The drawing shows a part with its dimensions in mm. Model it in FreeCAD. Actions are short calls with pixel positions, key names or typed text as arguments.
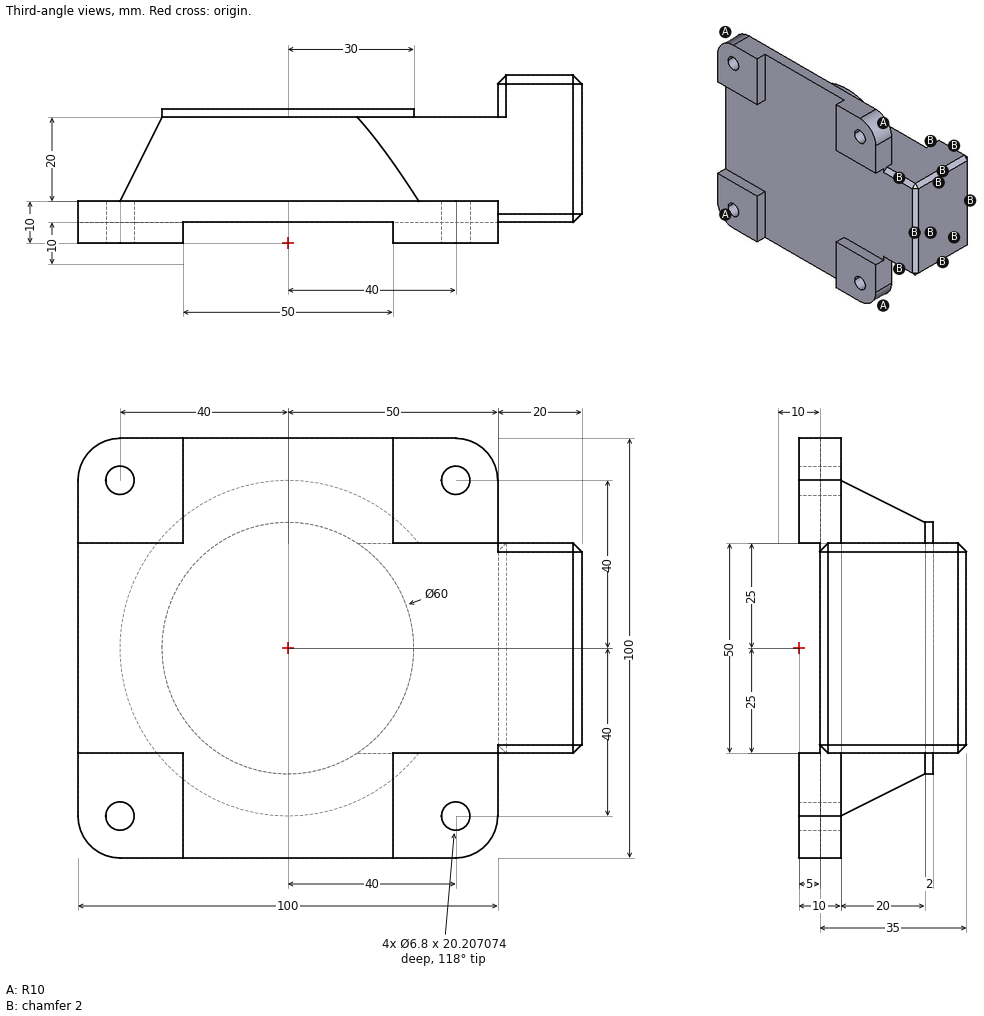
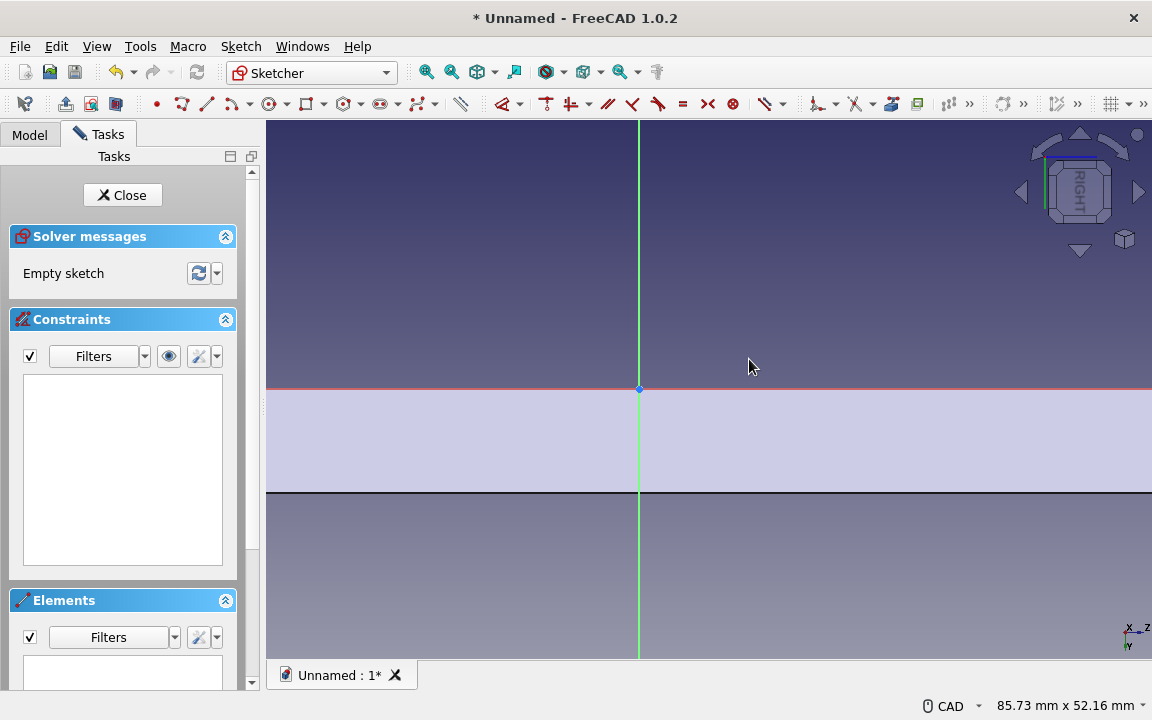
key(g)
key(v)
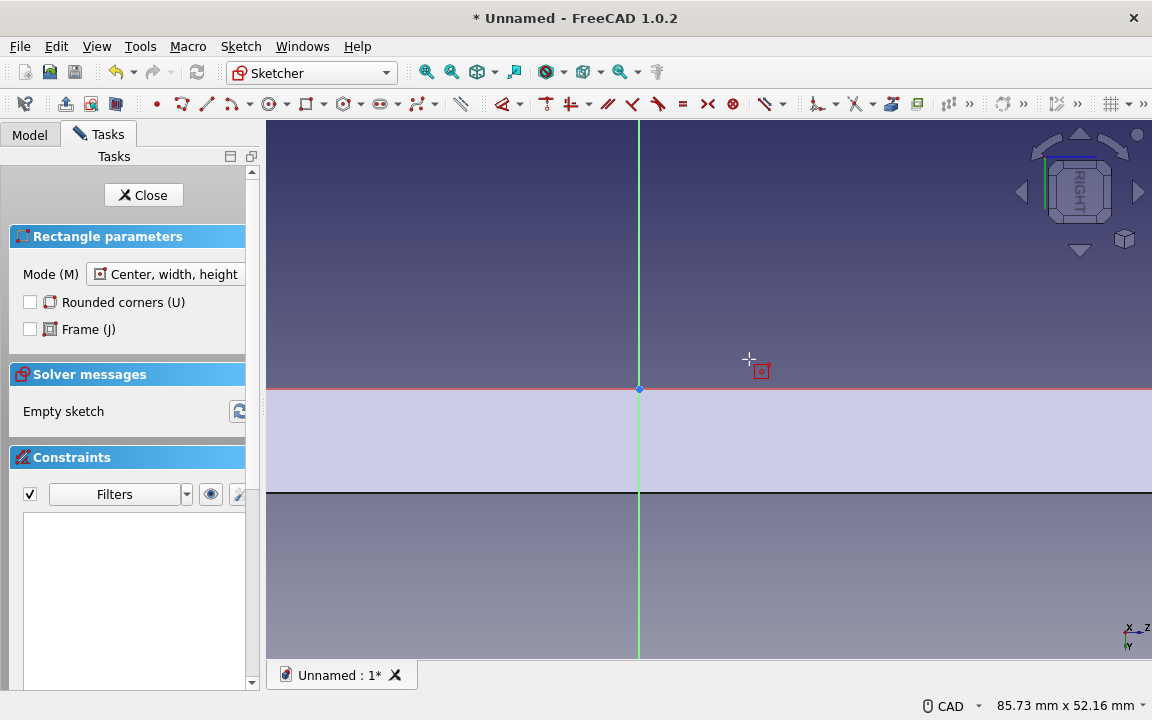
click(639, 389)
click(898, 338)
key(Escape)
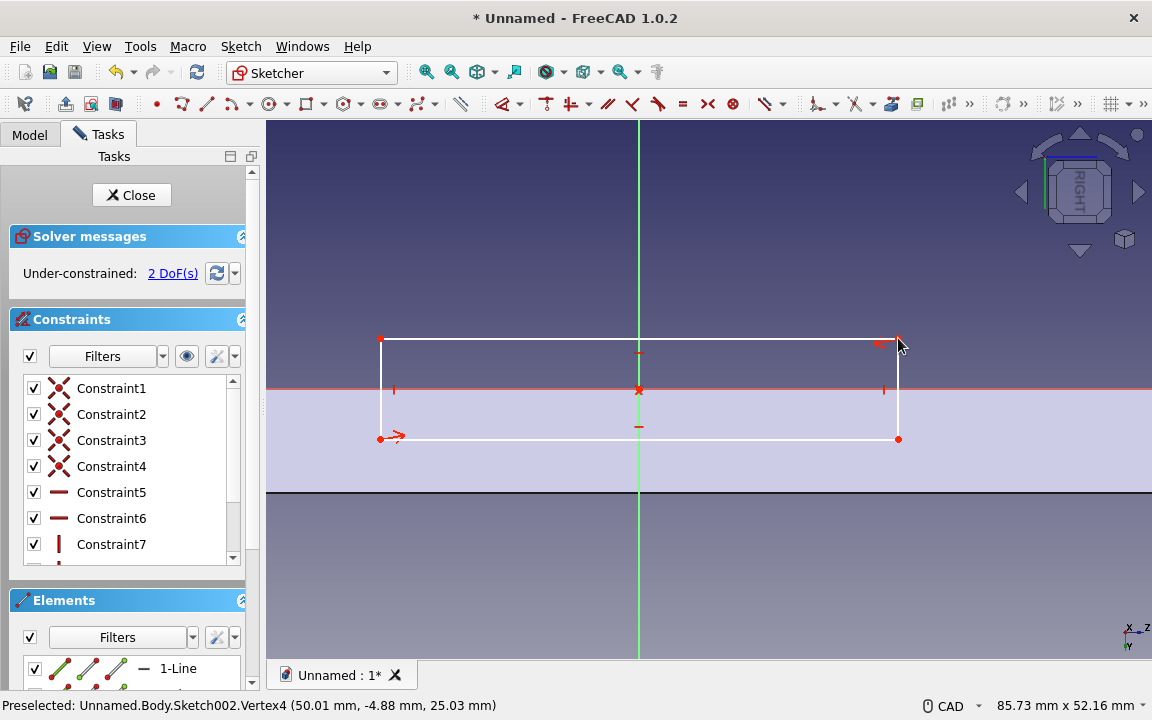
click(502, 104)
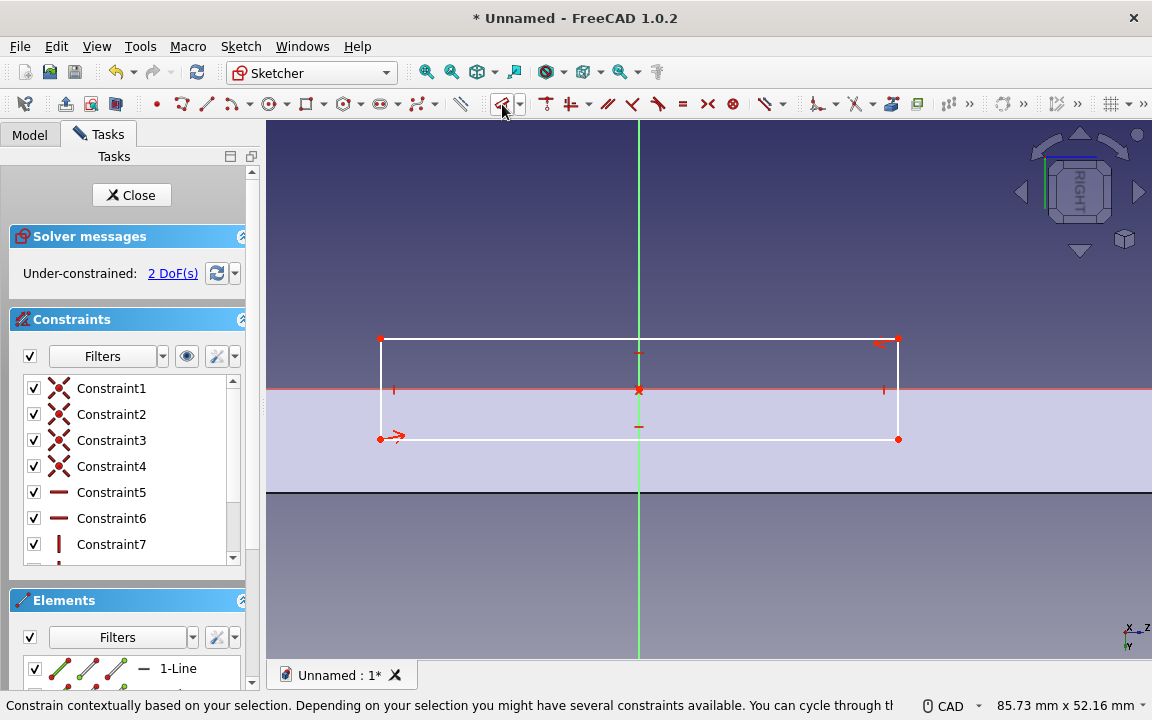
click(536, 440)
click(520, 474)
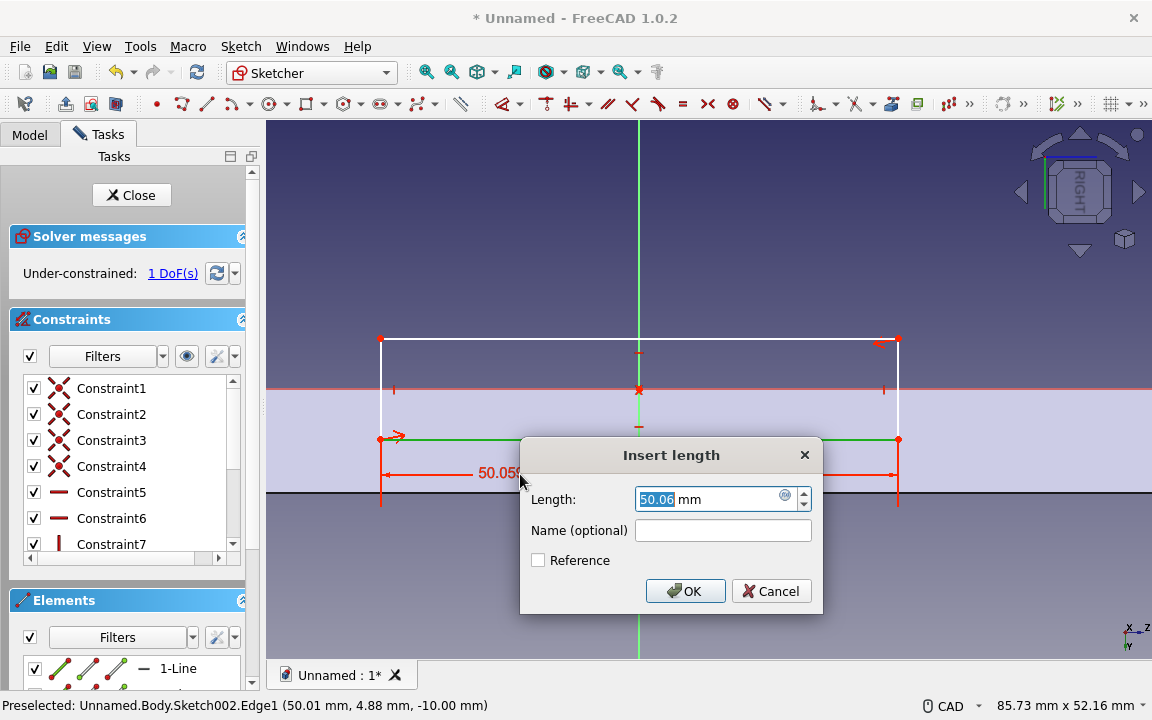
text(50)
key(Return)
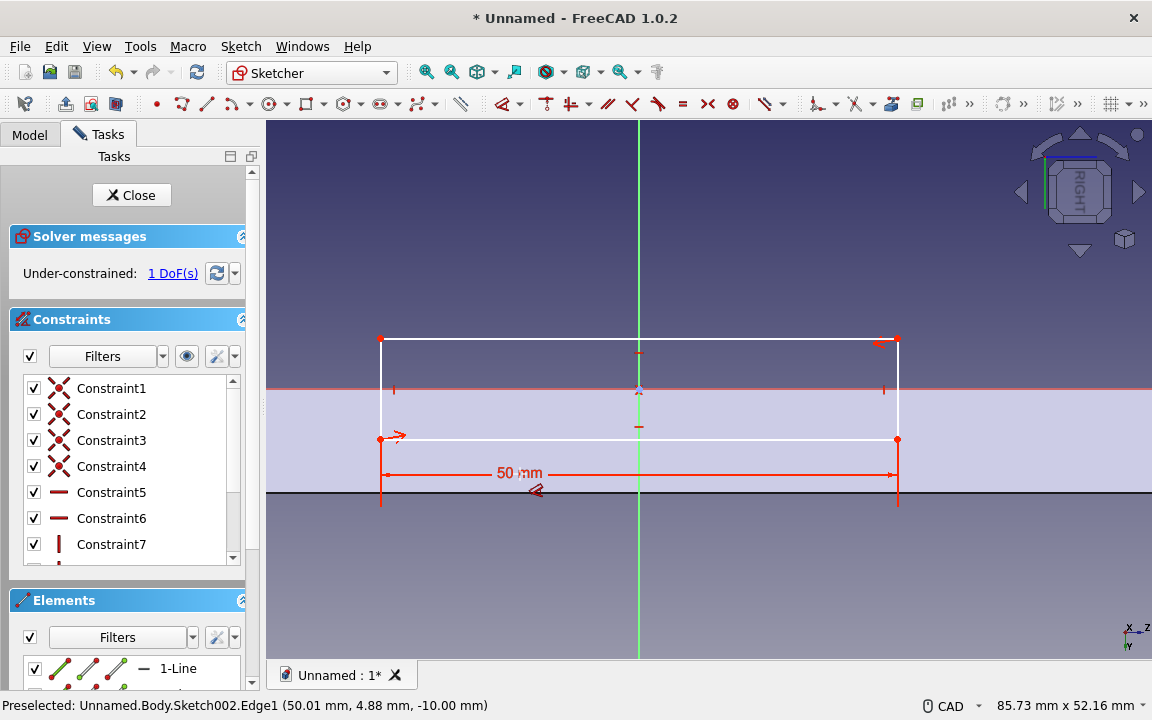
click(898, 410)
click(932, 366)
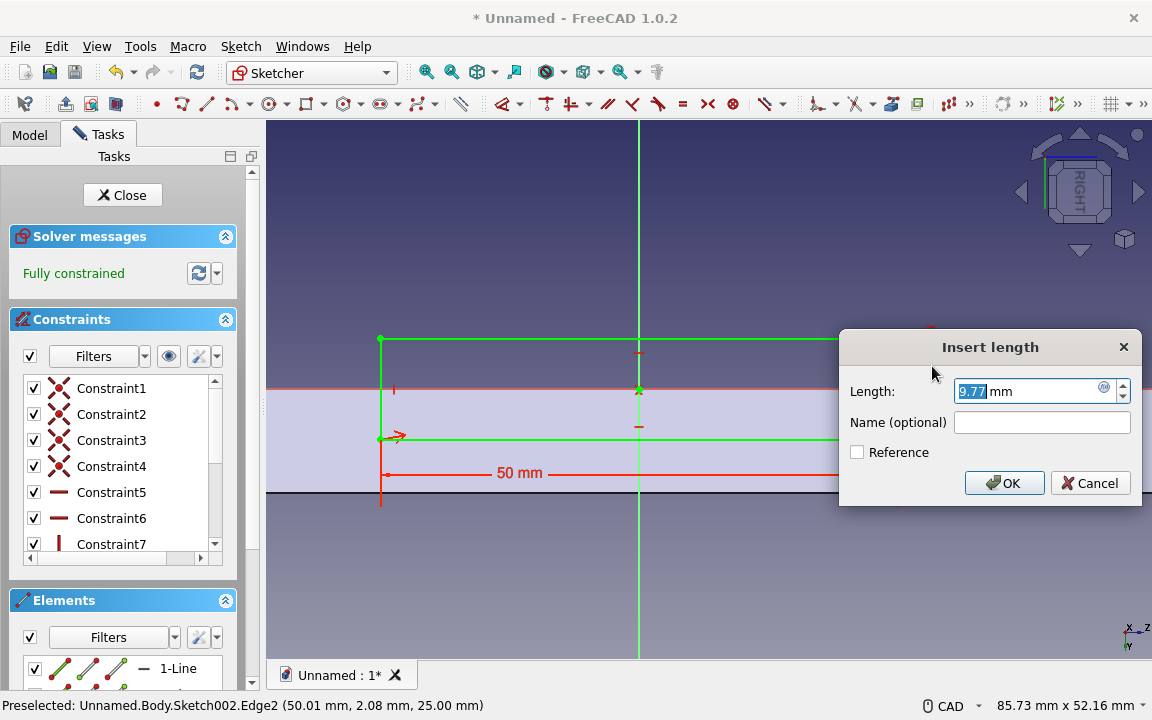
text(10)
key(Return)
key(Escape)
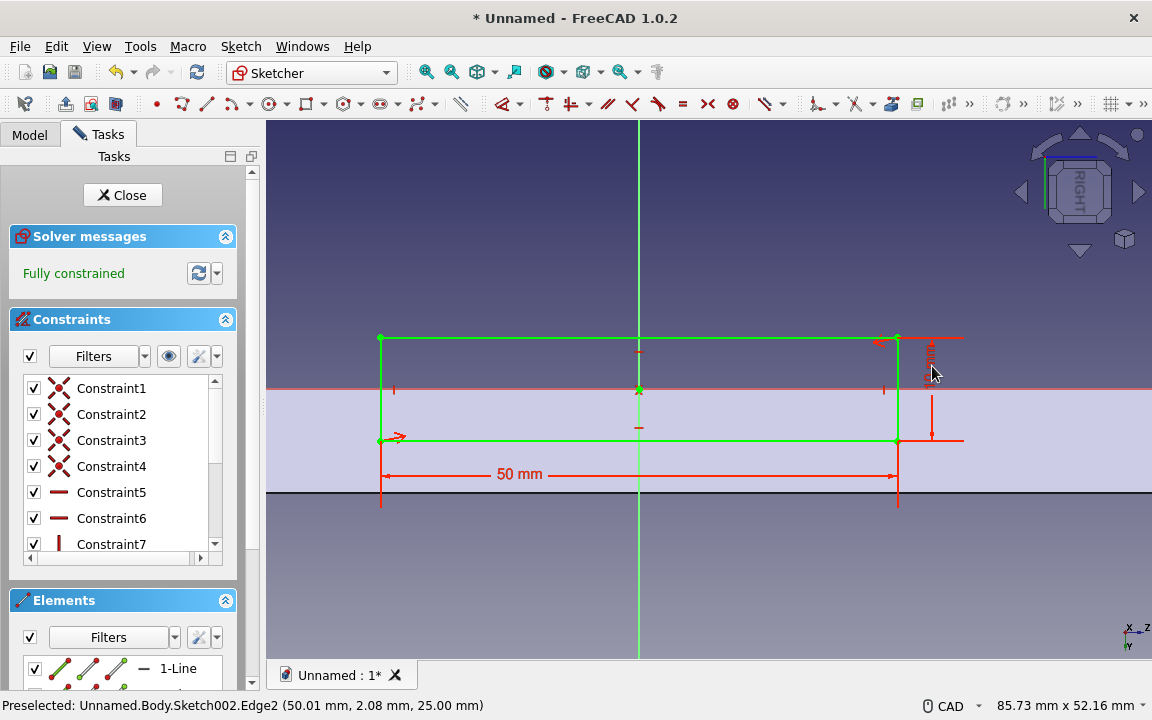
click(123, 195)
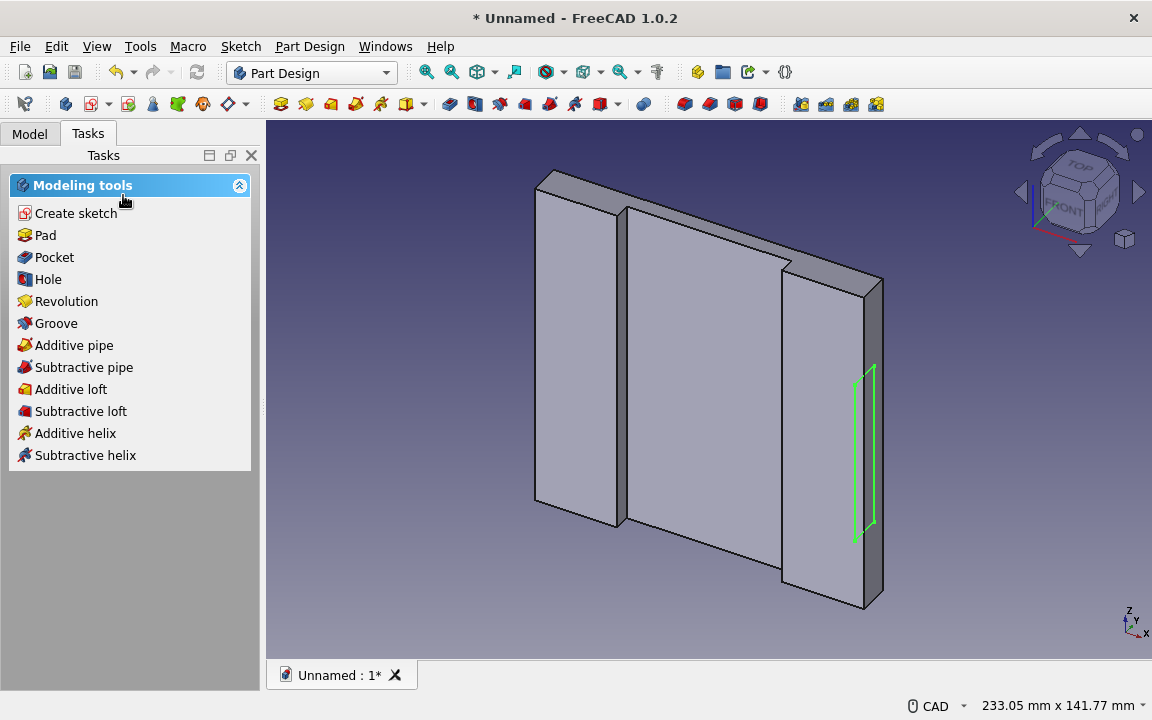
click(450, 104)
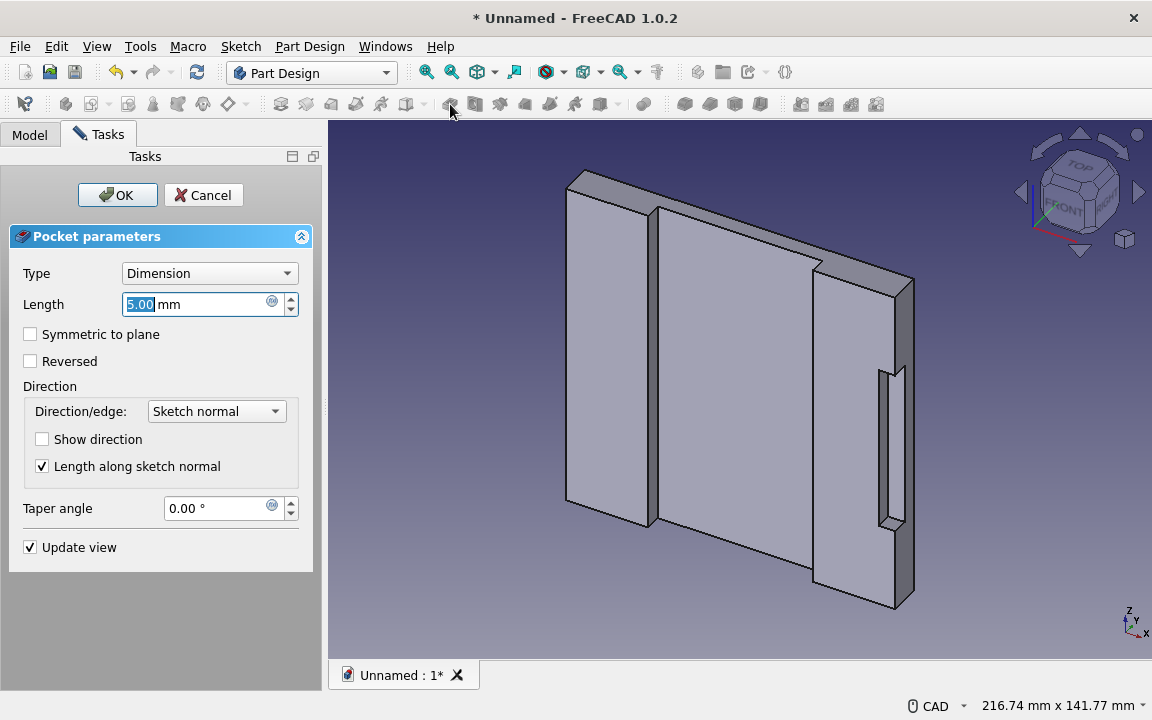
click(210, 274)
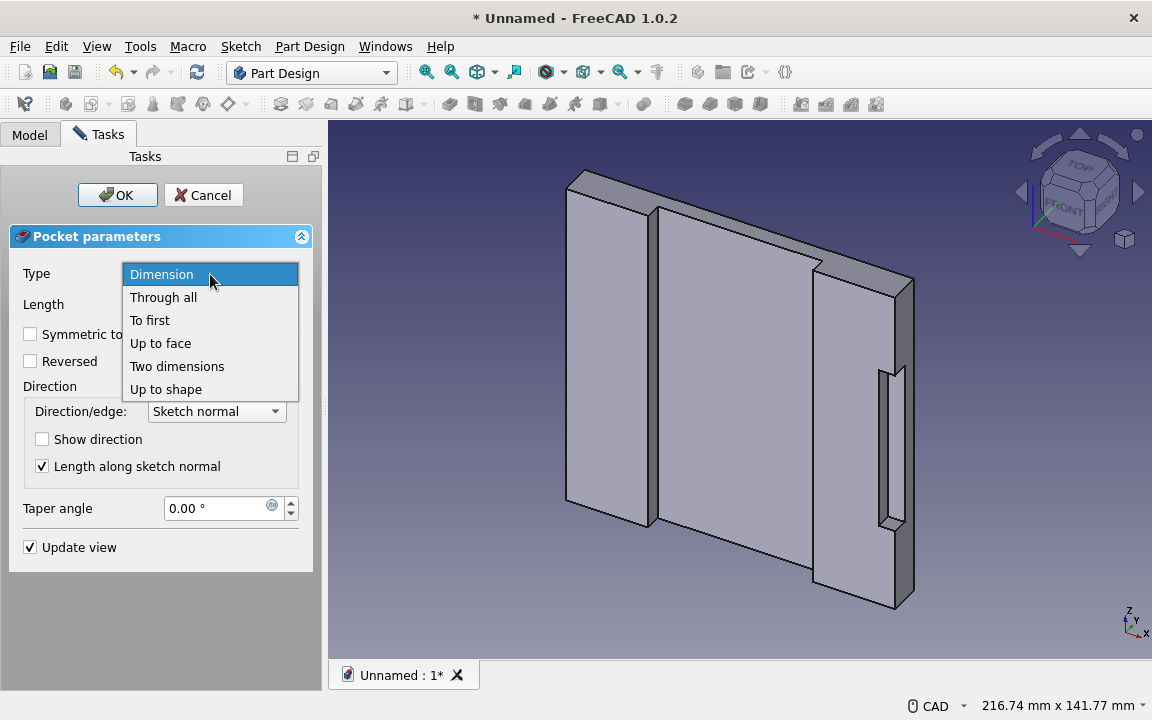
click(208, 298)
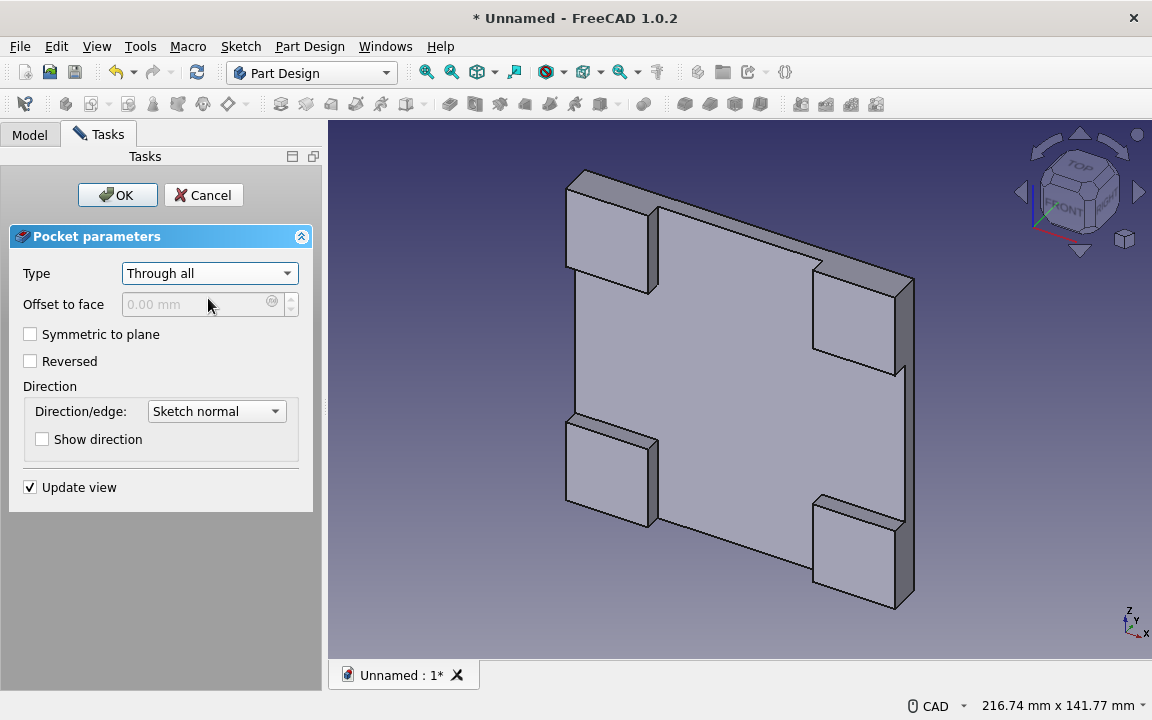
click(118, 195)